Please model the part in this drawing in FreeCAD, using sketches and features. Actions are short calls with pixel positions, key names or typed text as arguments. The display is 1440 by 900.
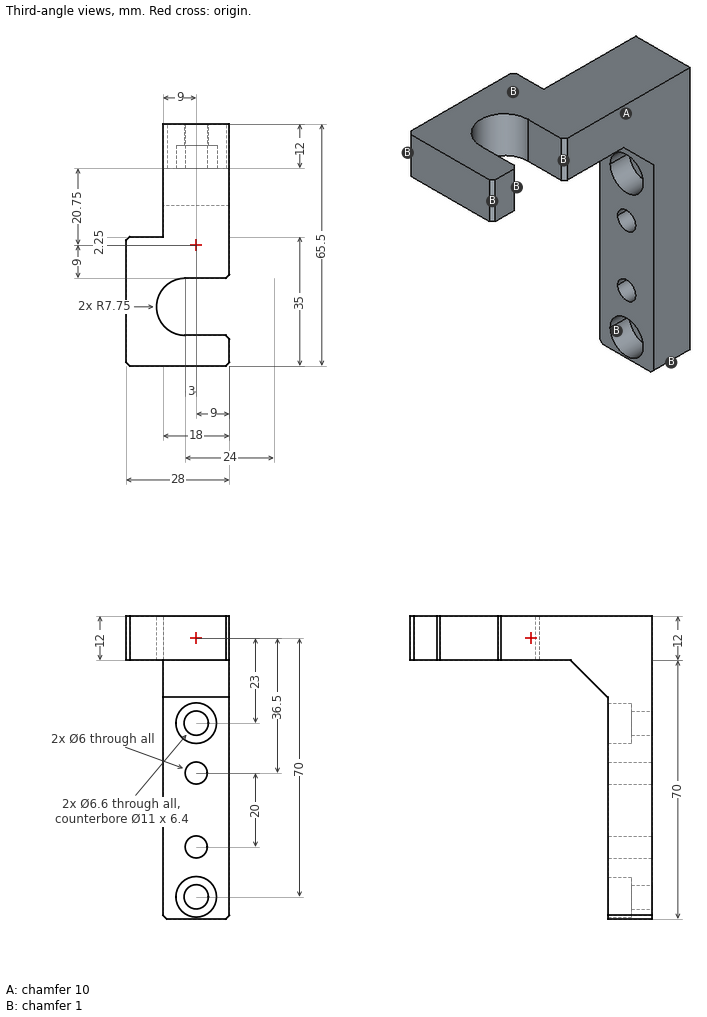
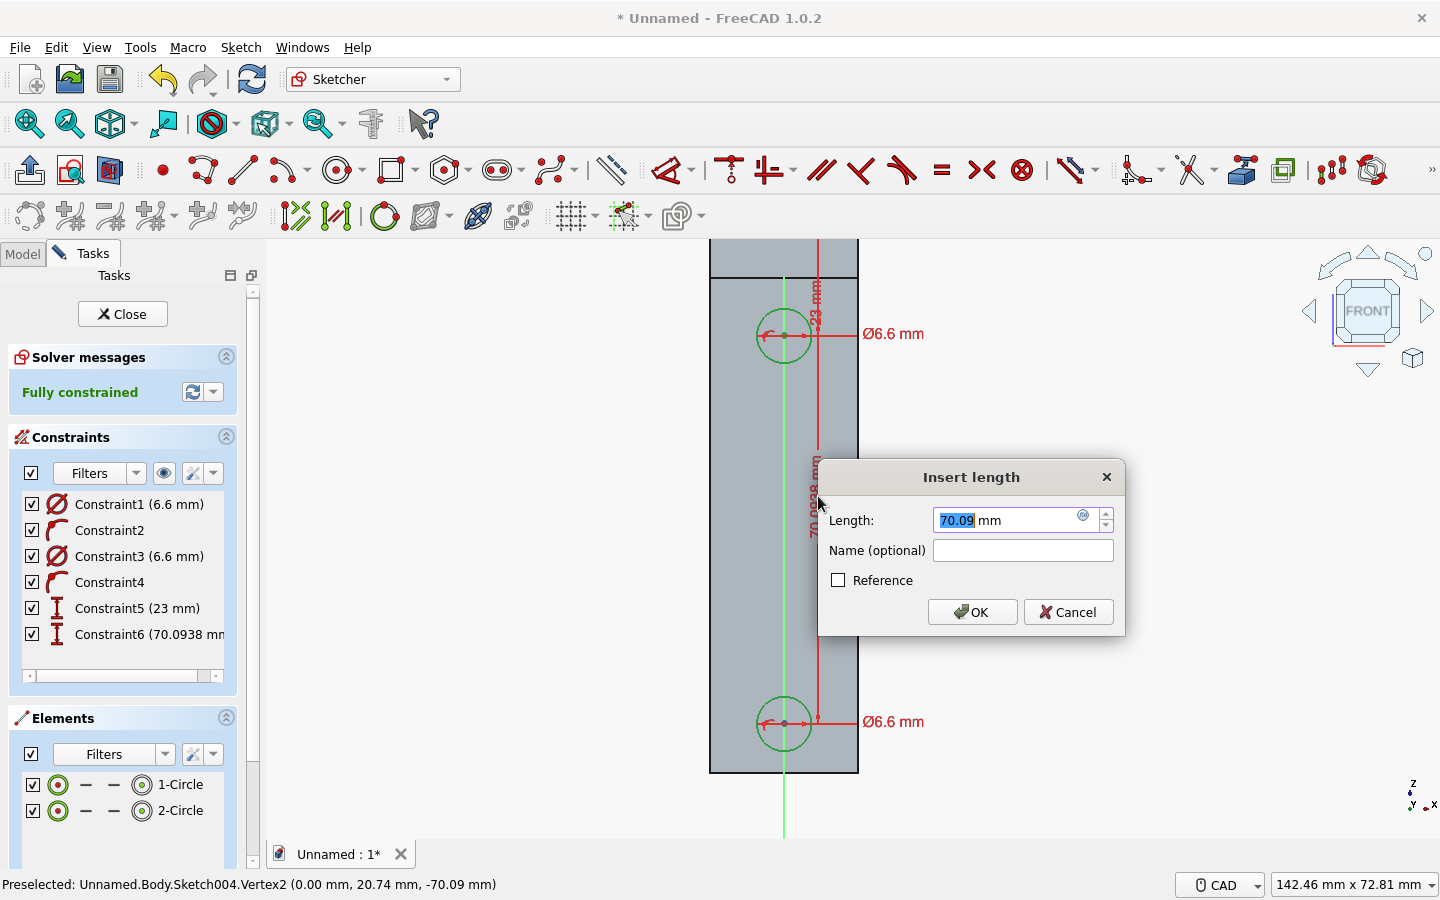
text(70)
key(Return)
key(Escape)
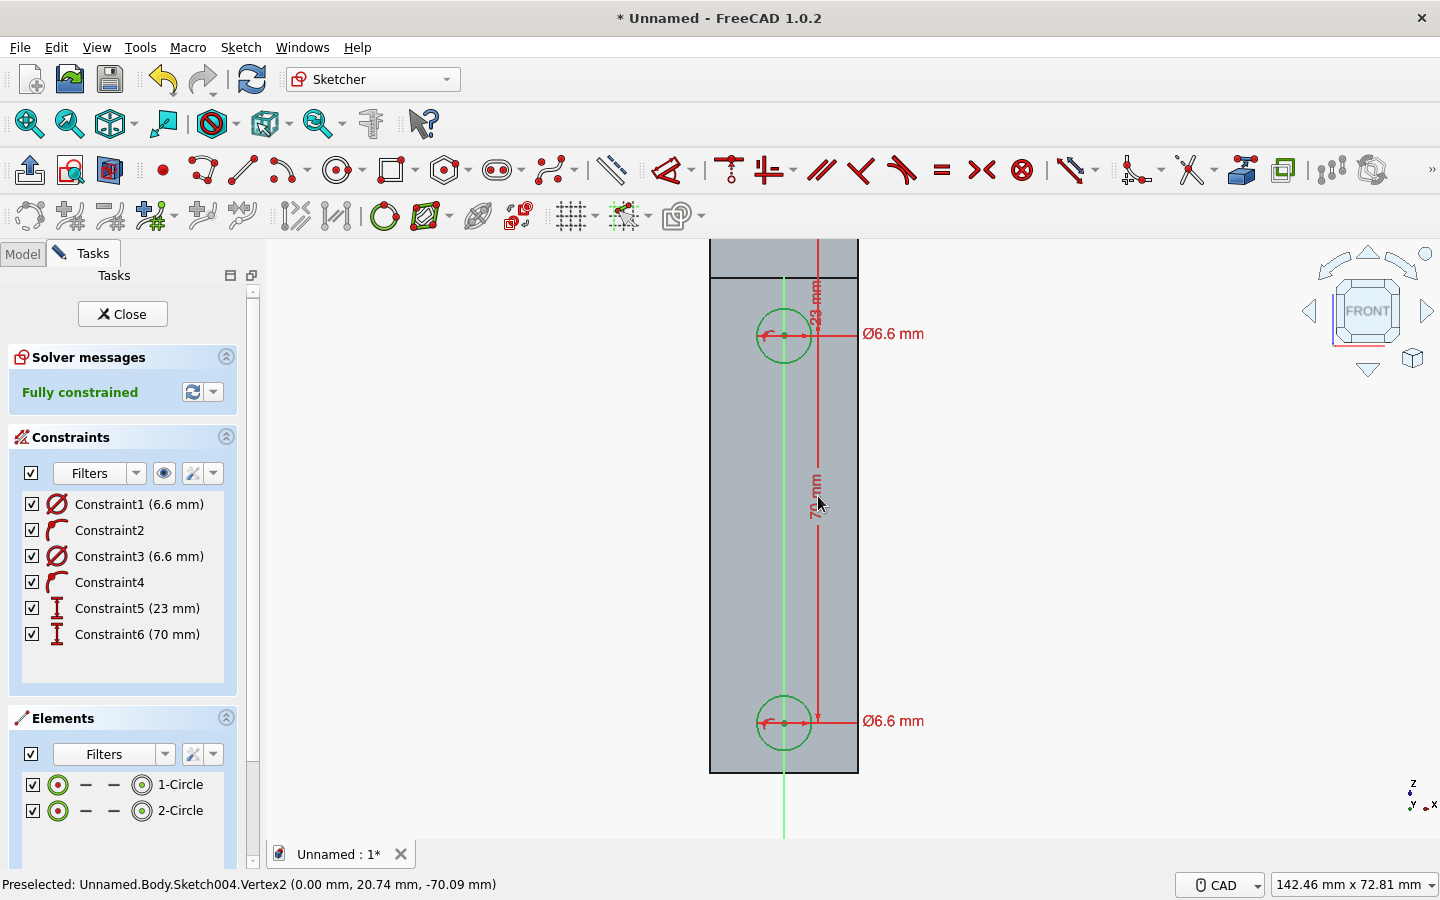
click(123, 314)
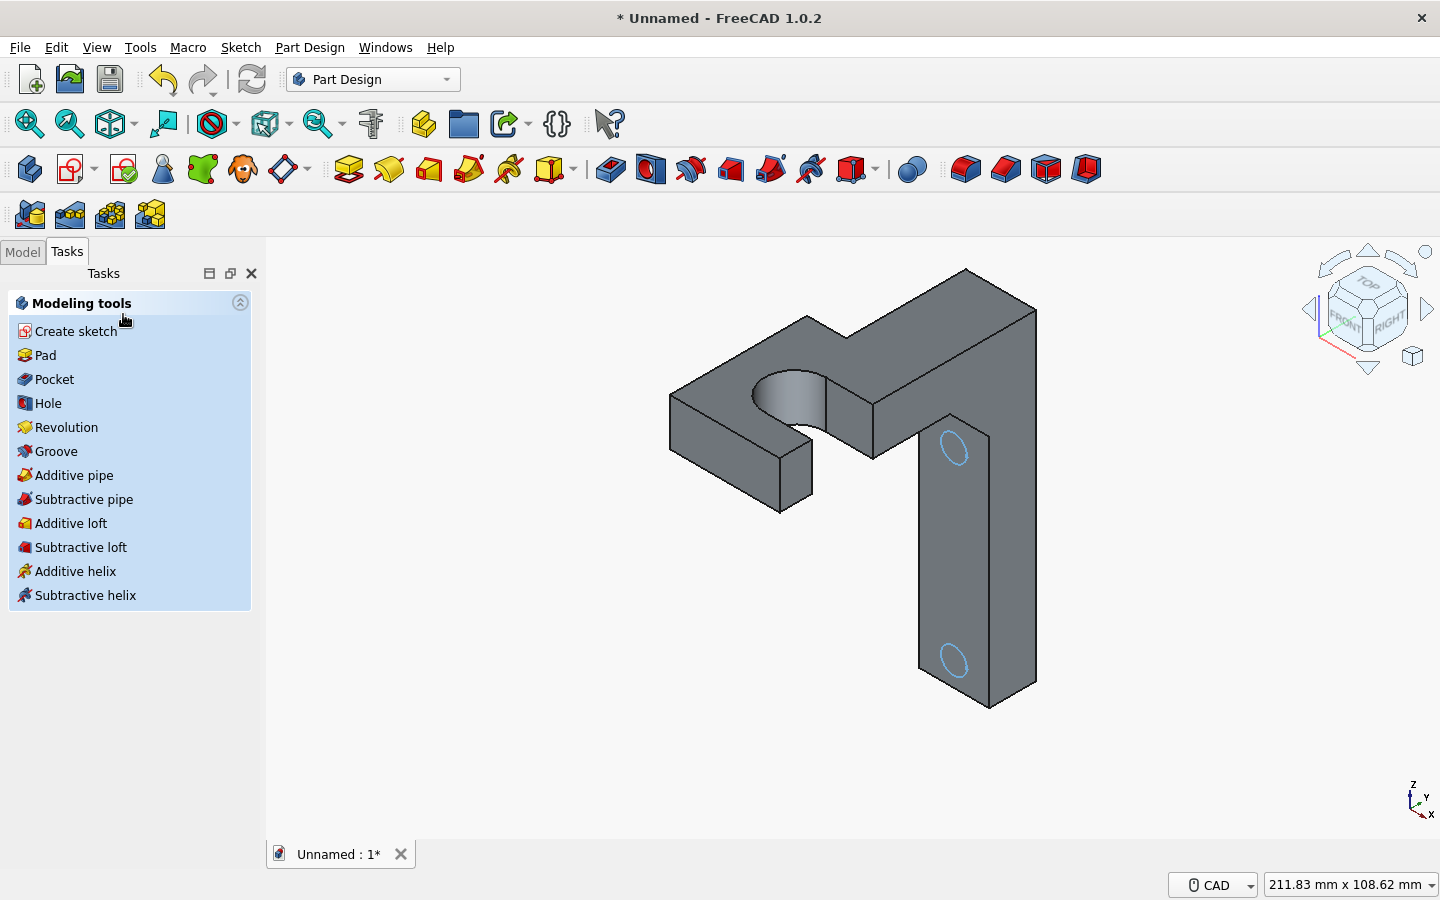
click(652, 170)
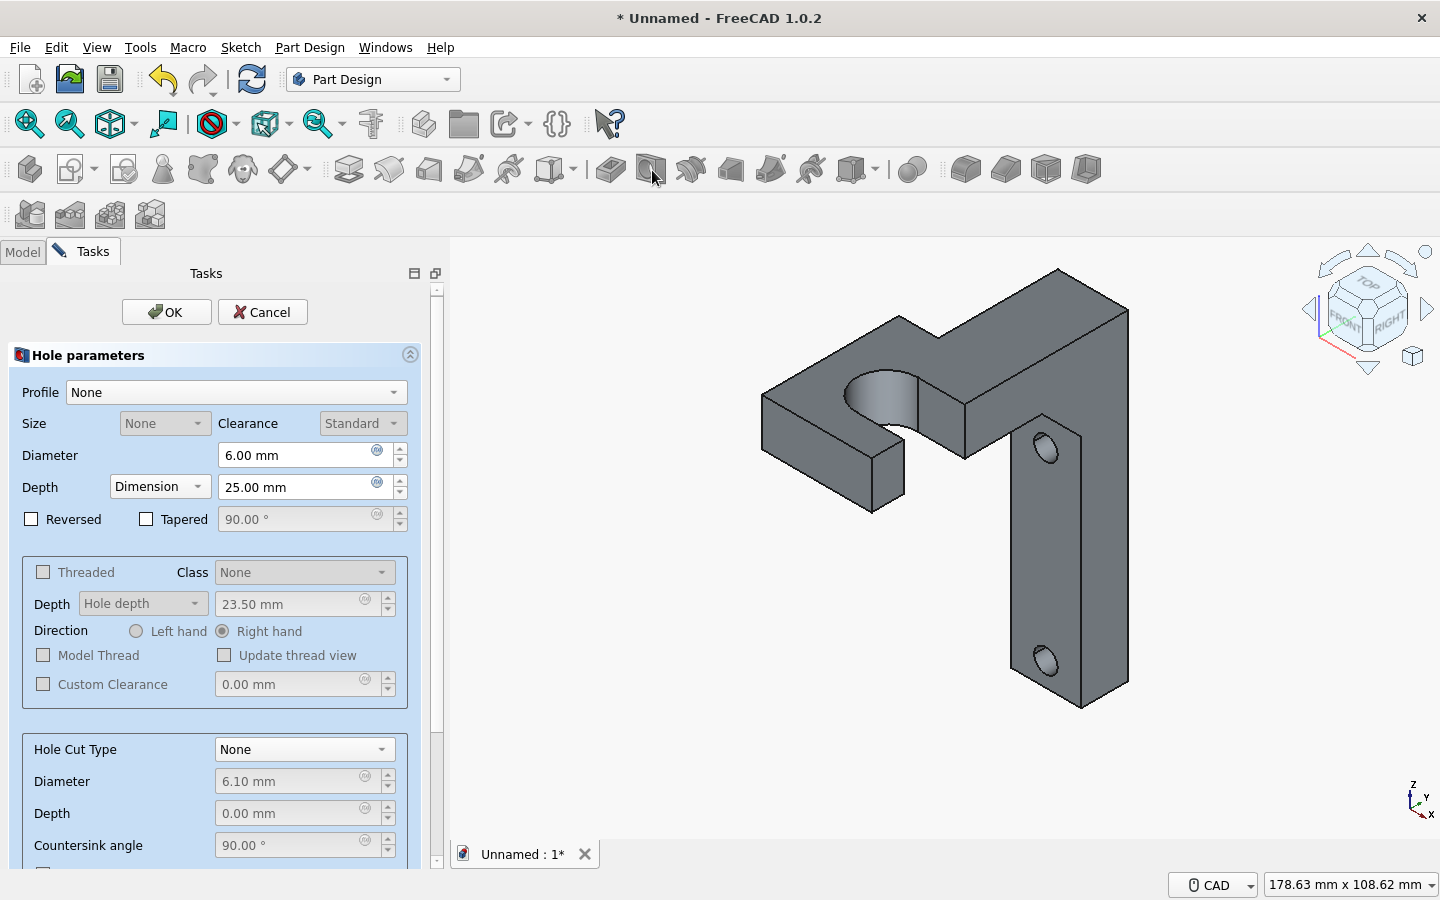
triple_click(305, 455)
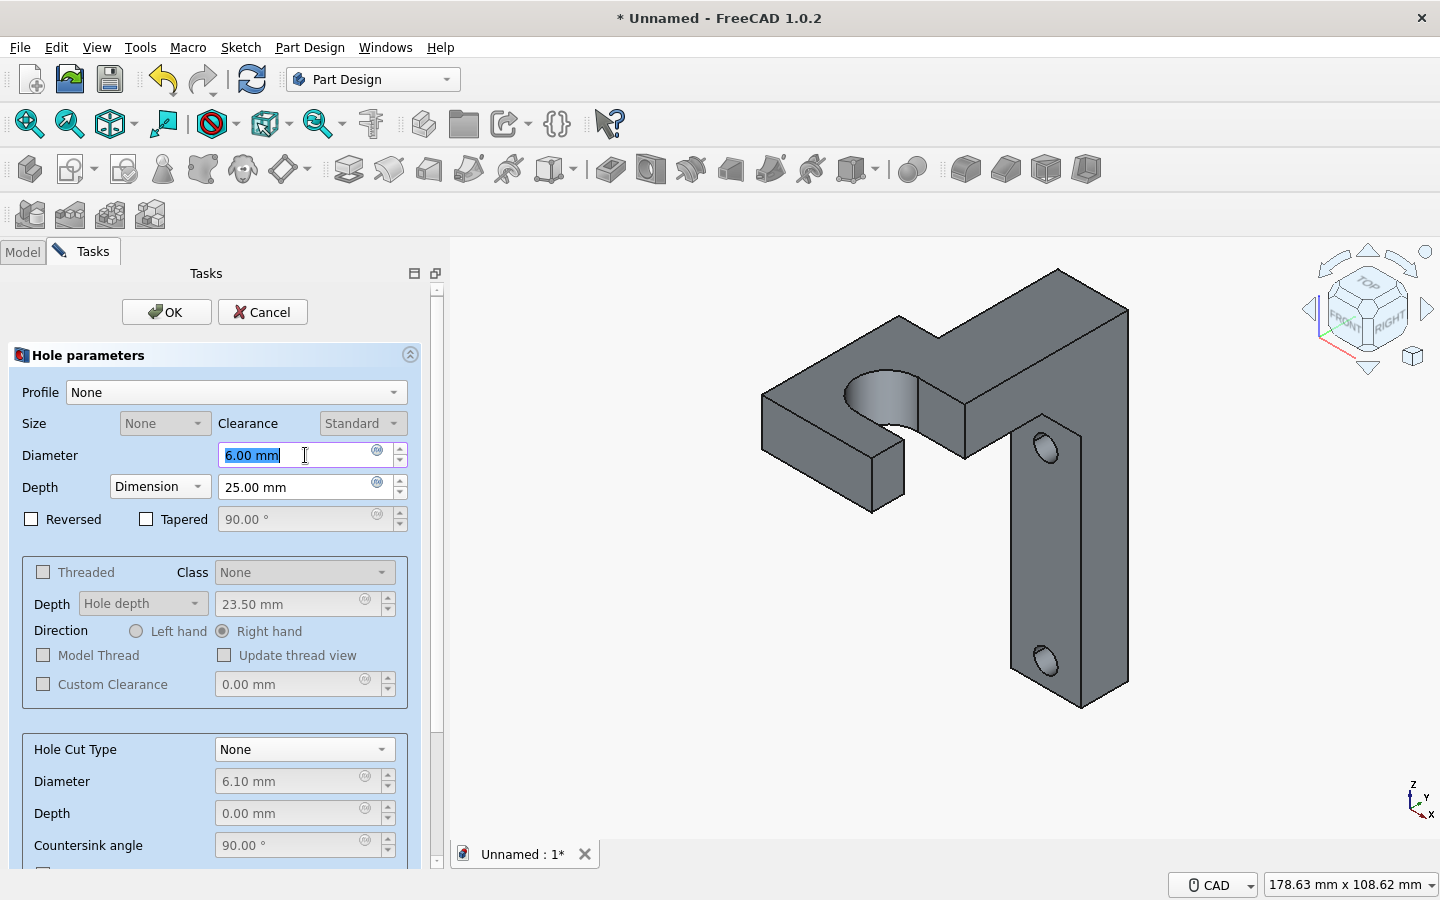
text(6.6)
key(Tab)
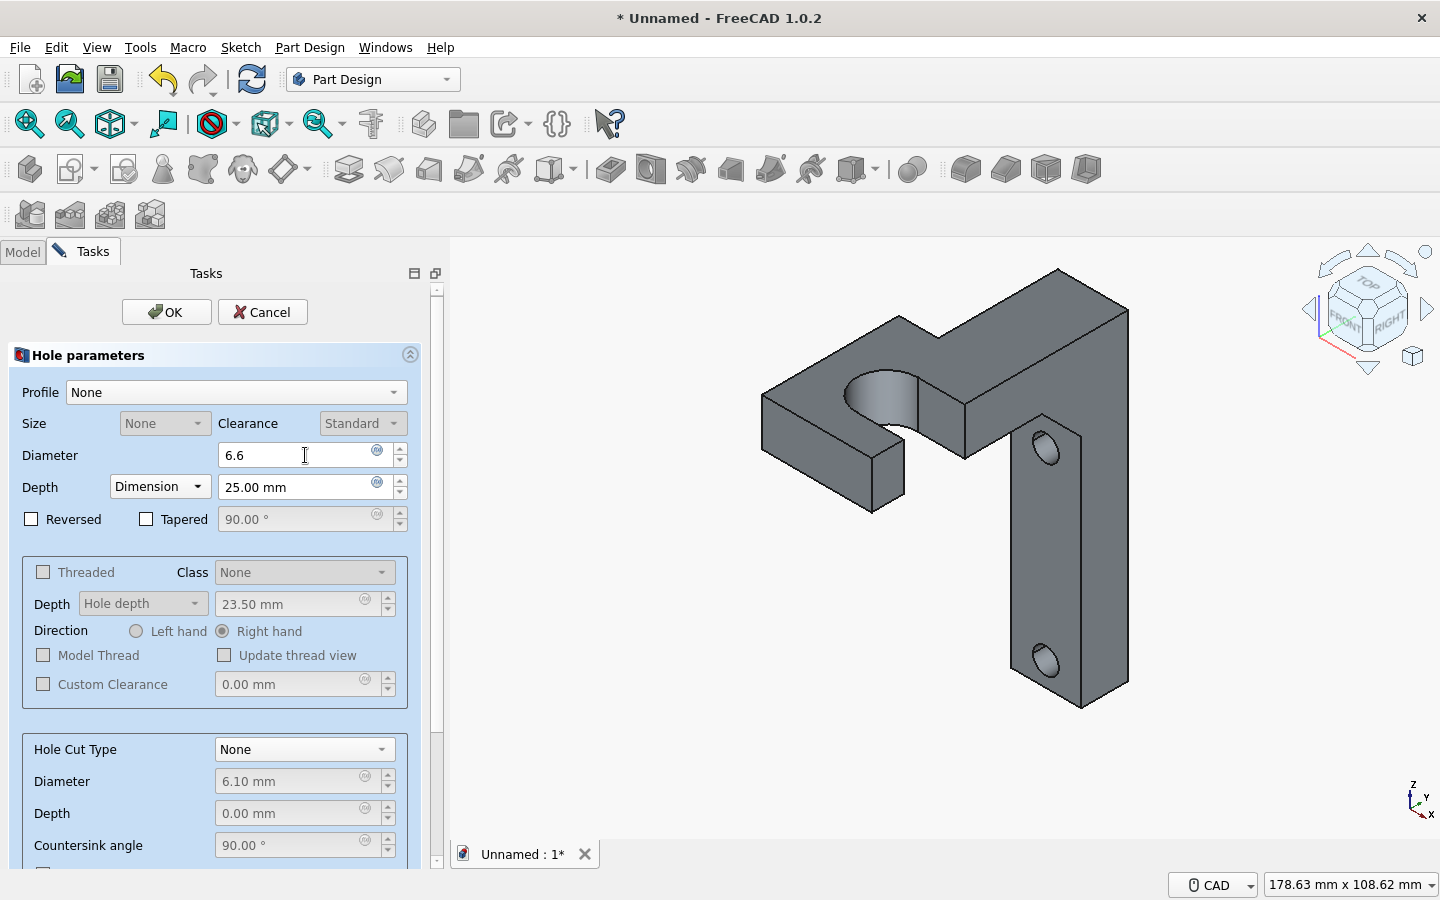
click(161, 486)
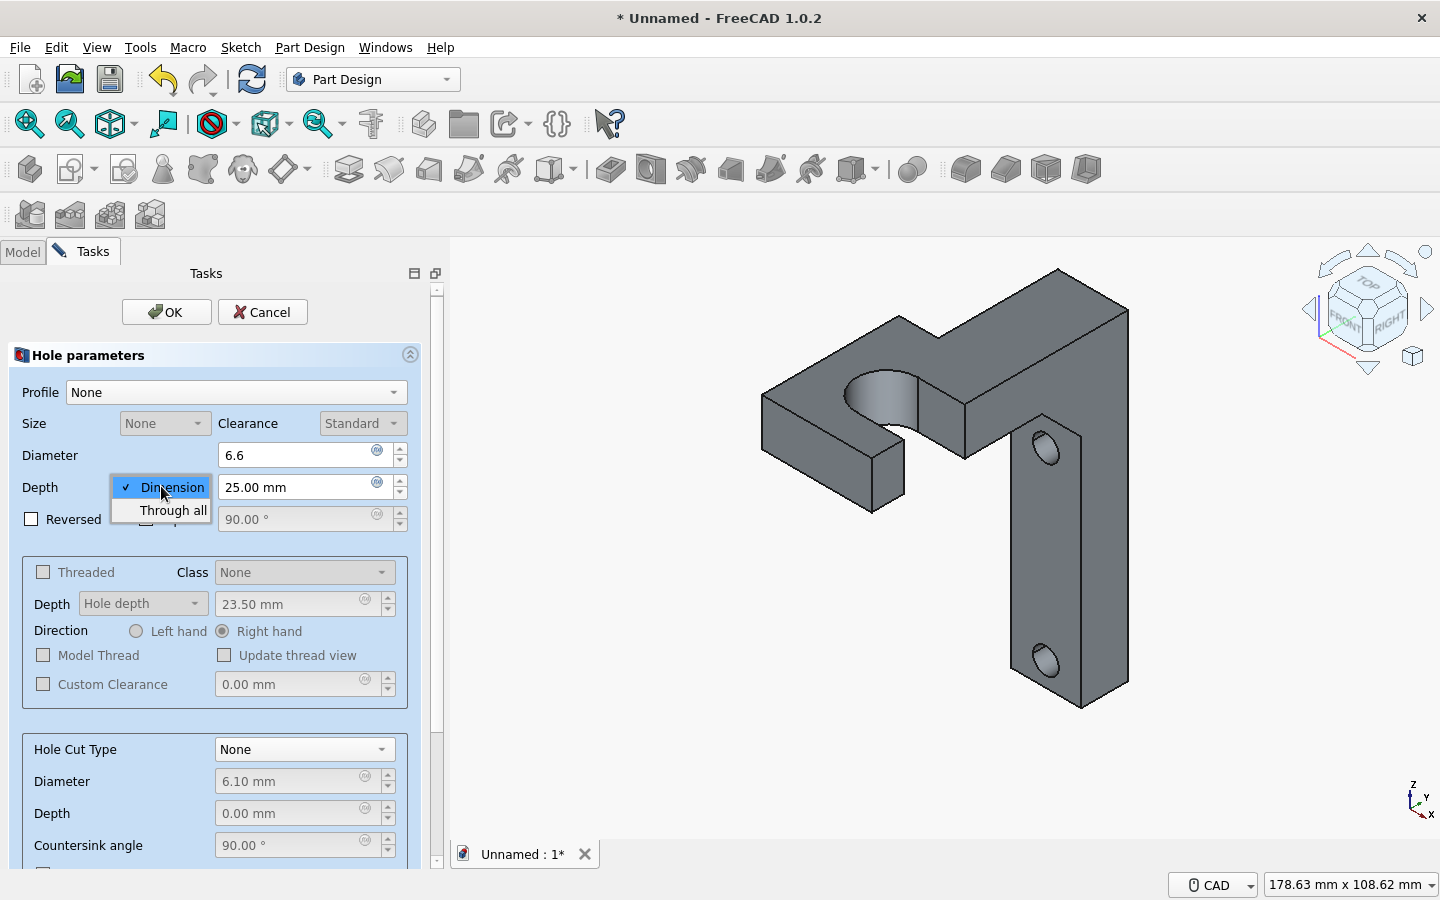
click(160, 510)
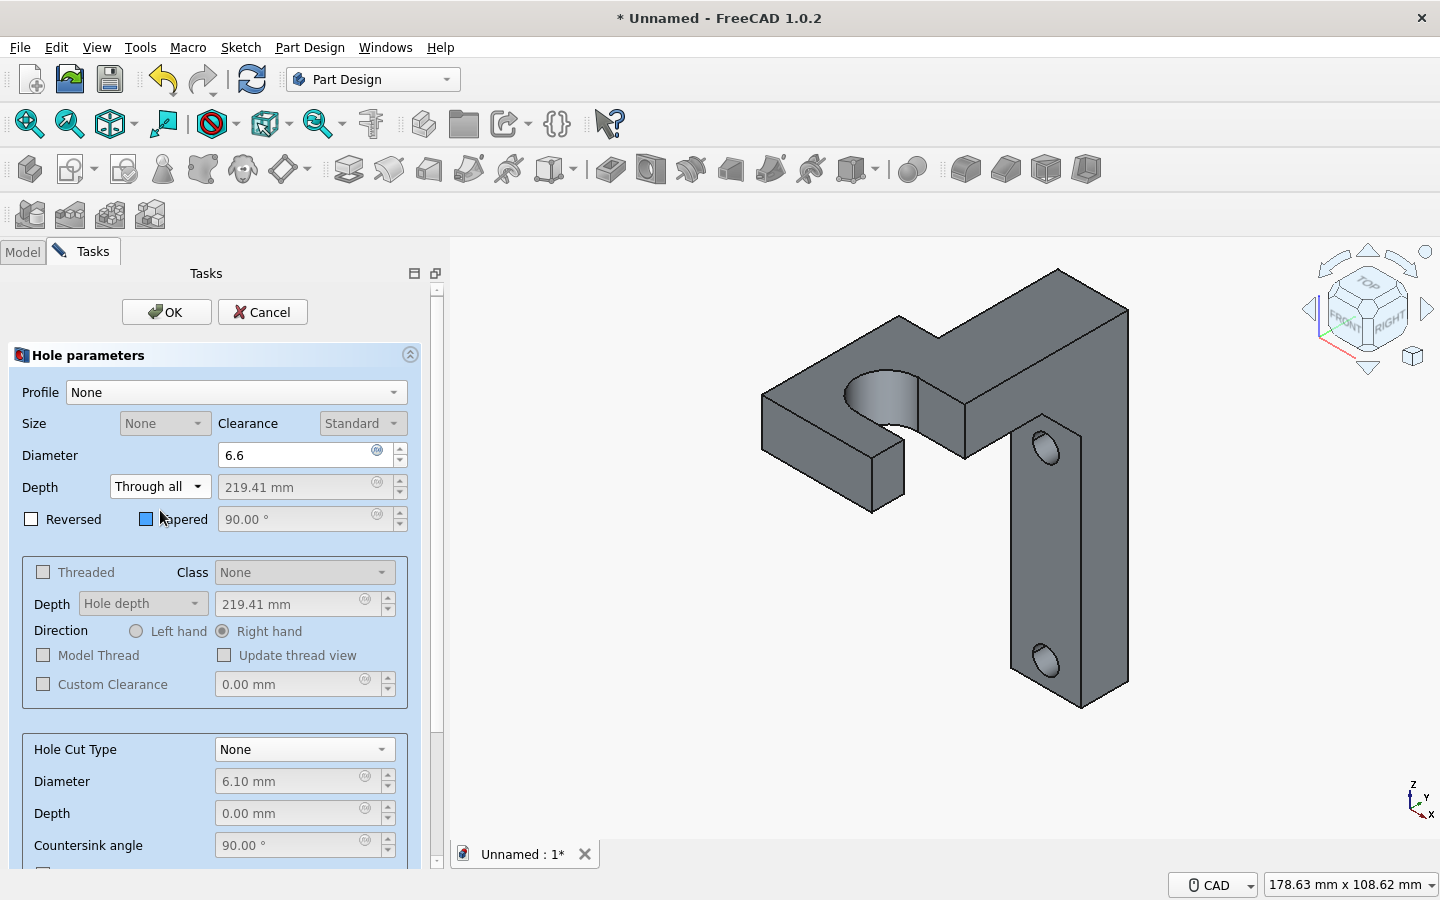
click(306, 750)